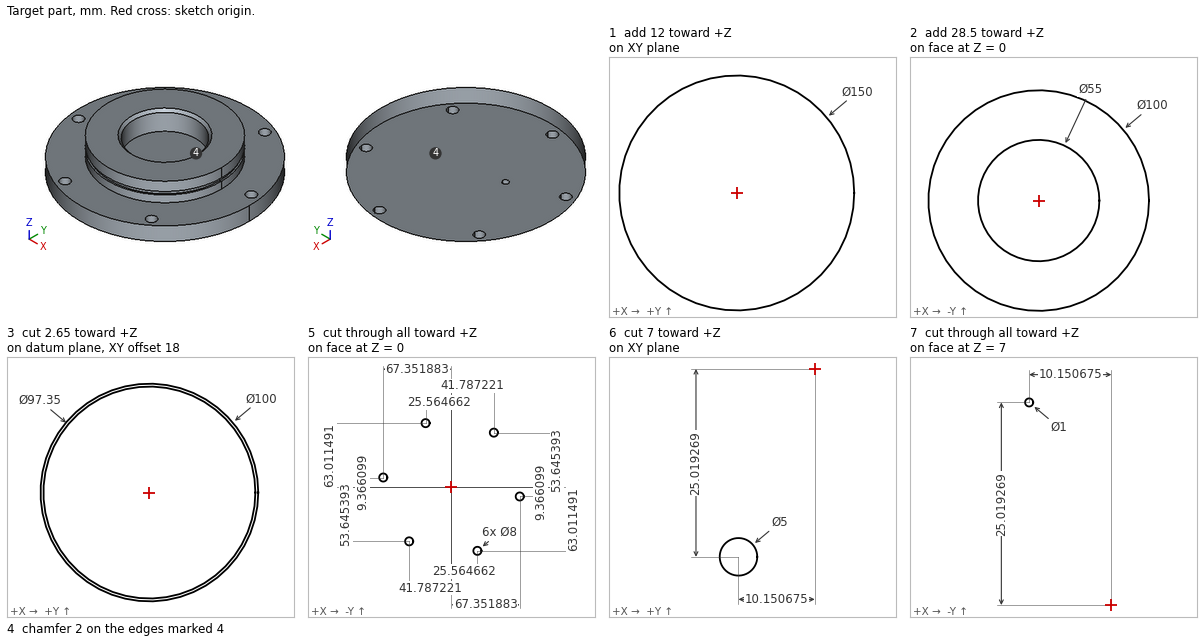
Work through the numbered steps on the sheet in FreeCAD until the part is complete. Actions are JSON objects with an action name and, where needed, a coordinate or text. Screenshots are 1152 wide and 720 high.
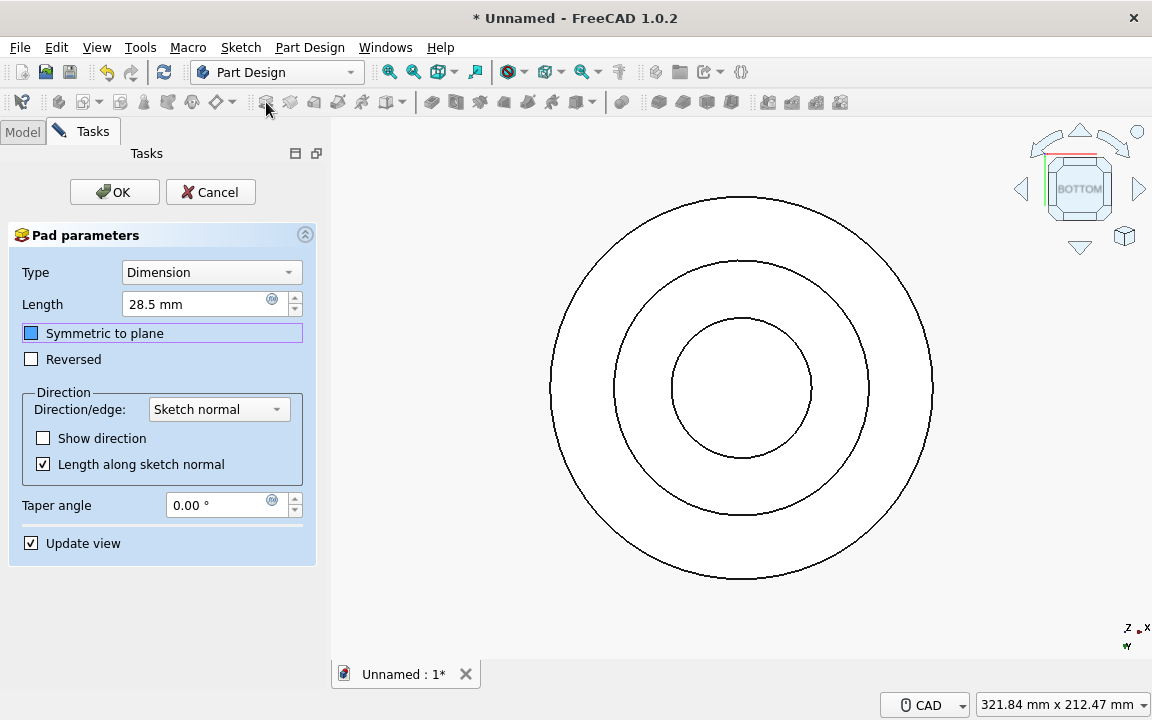
{"action": "left_click", "coordinate": [30, 359]}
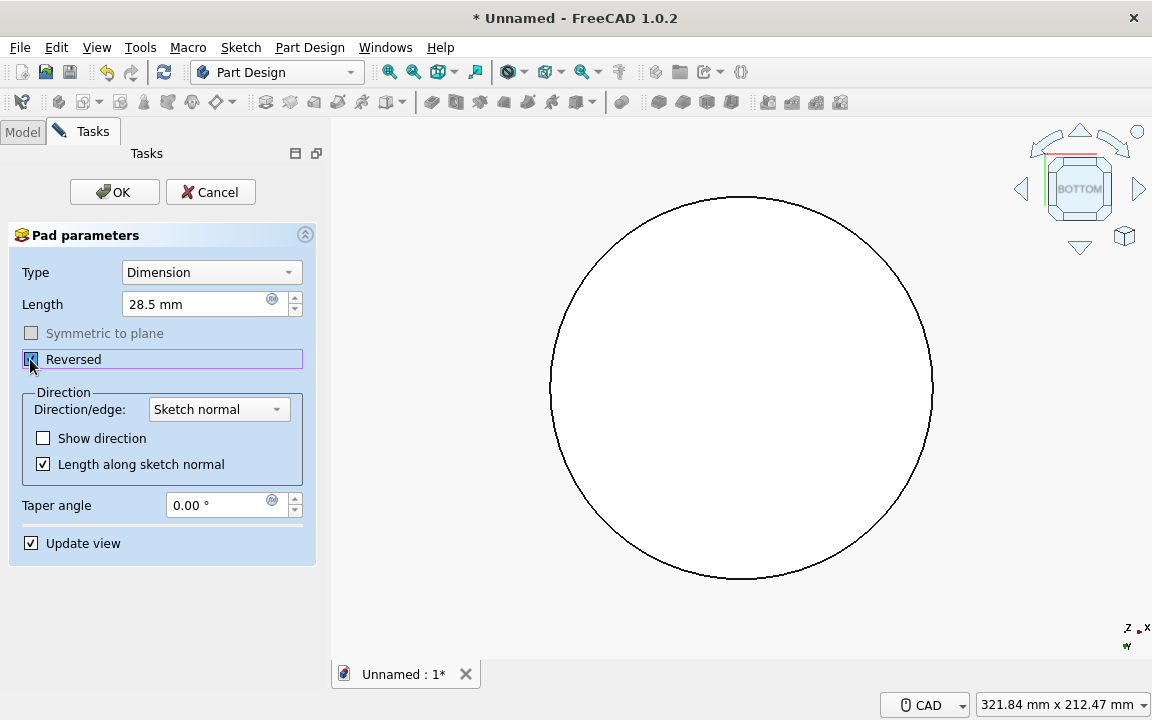
{"action": "left_click", "coordinate": [115, 192]}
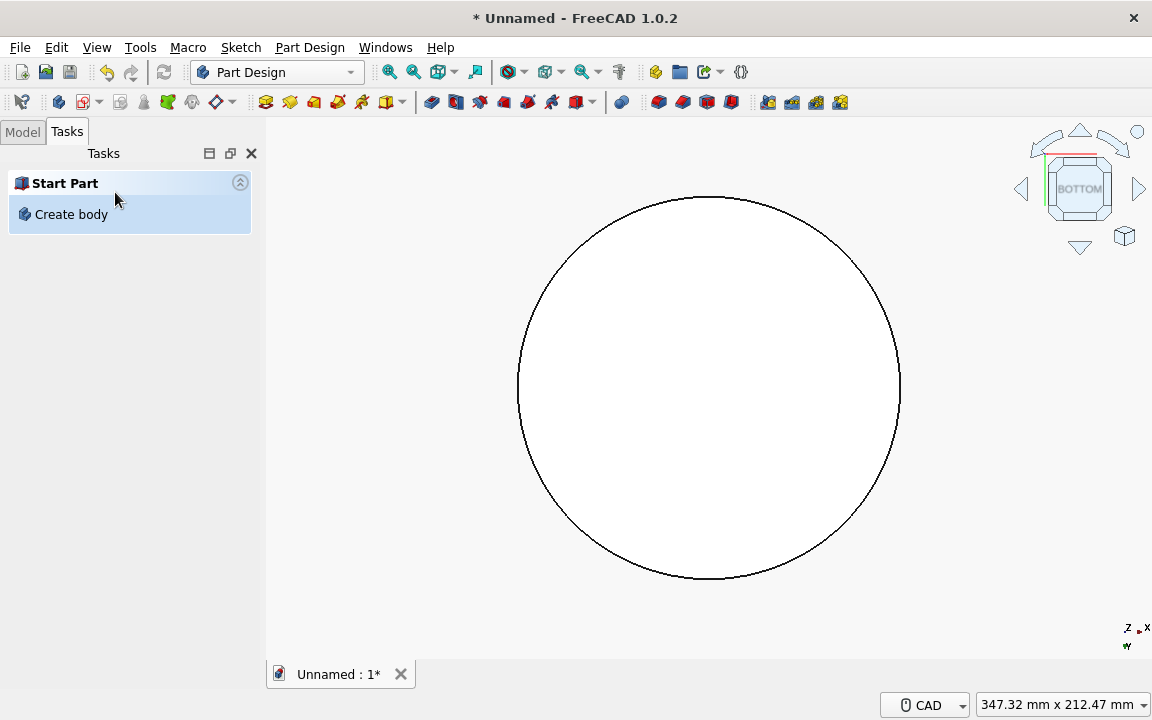
{"action": "left_click", "coordinate": [23, 131]}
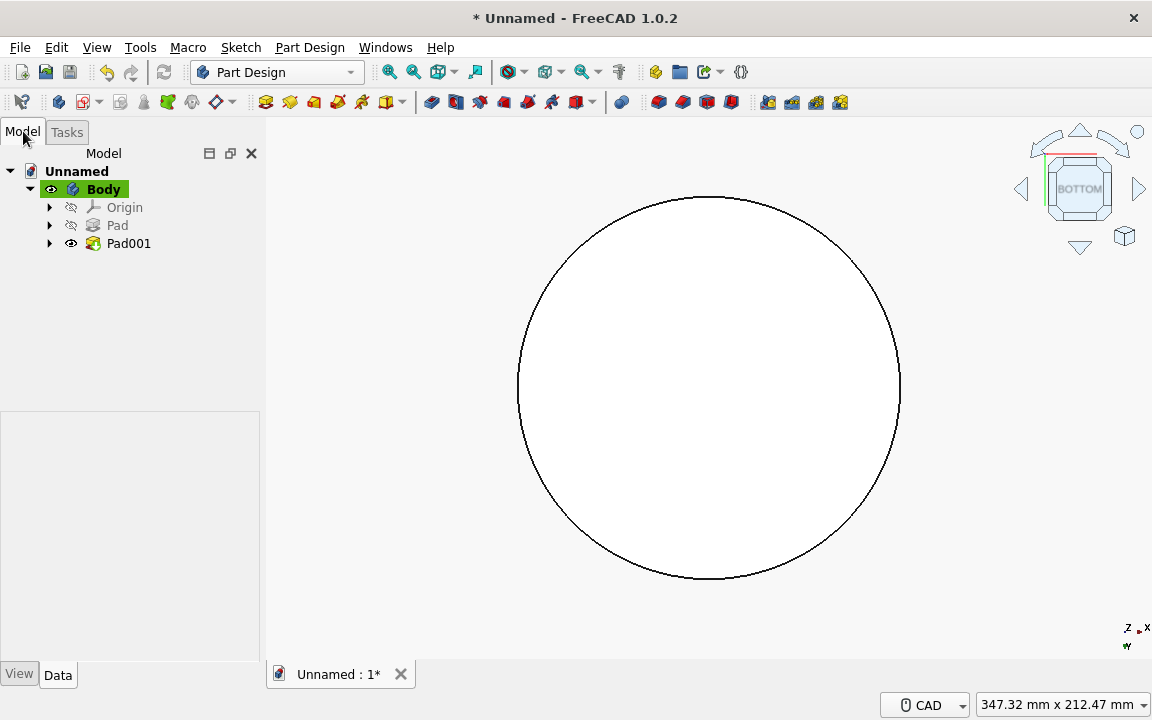
{"action": "left_click", "coordinate": [50, 207]}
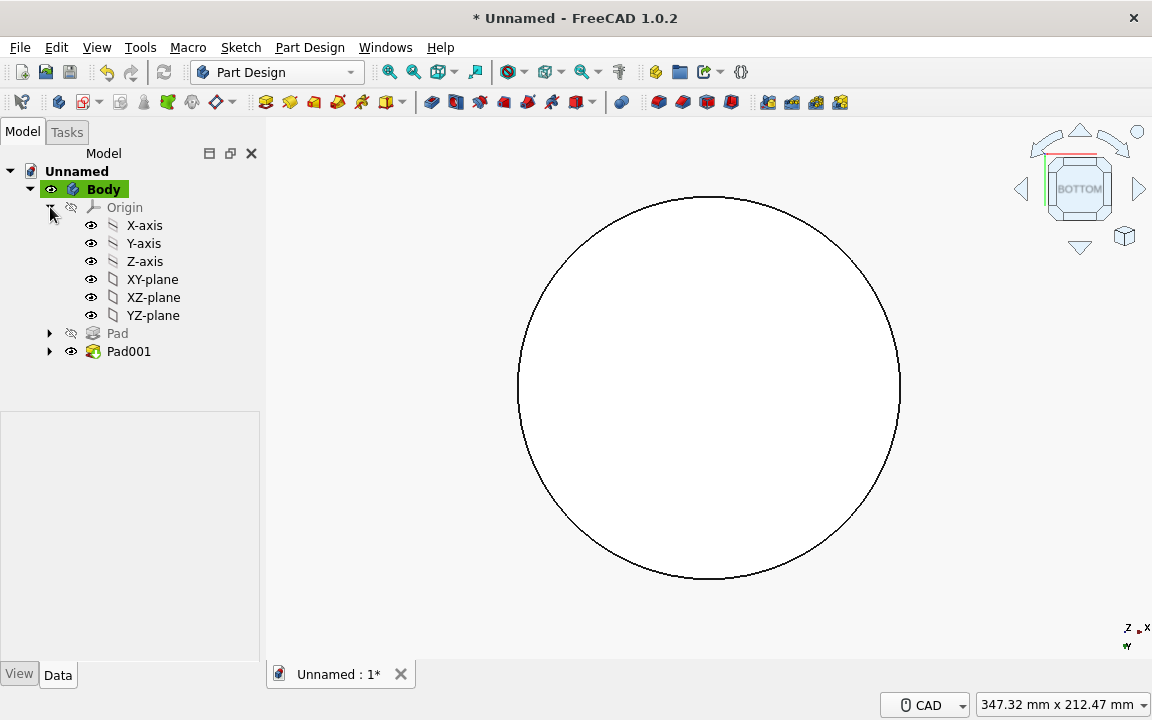
{"action": "left_click", "coordinate": [136, 279]}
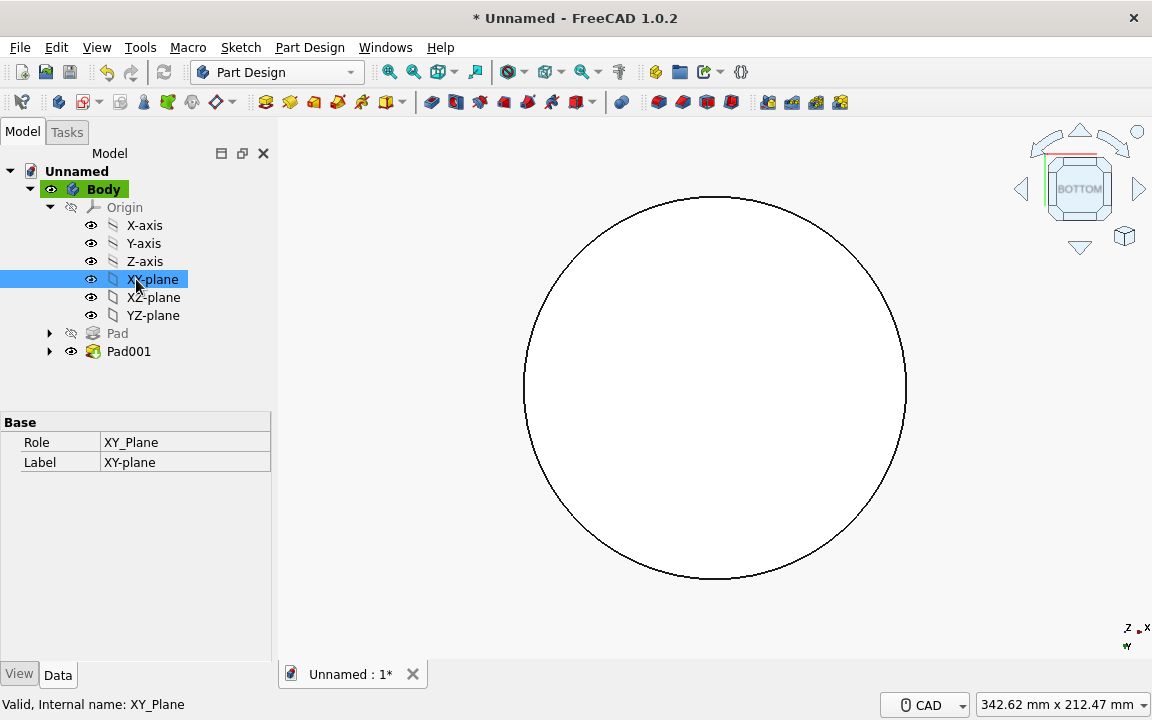
{"action": "left_click", "coordinate": [216, 102]}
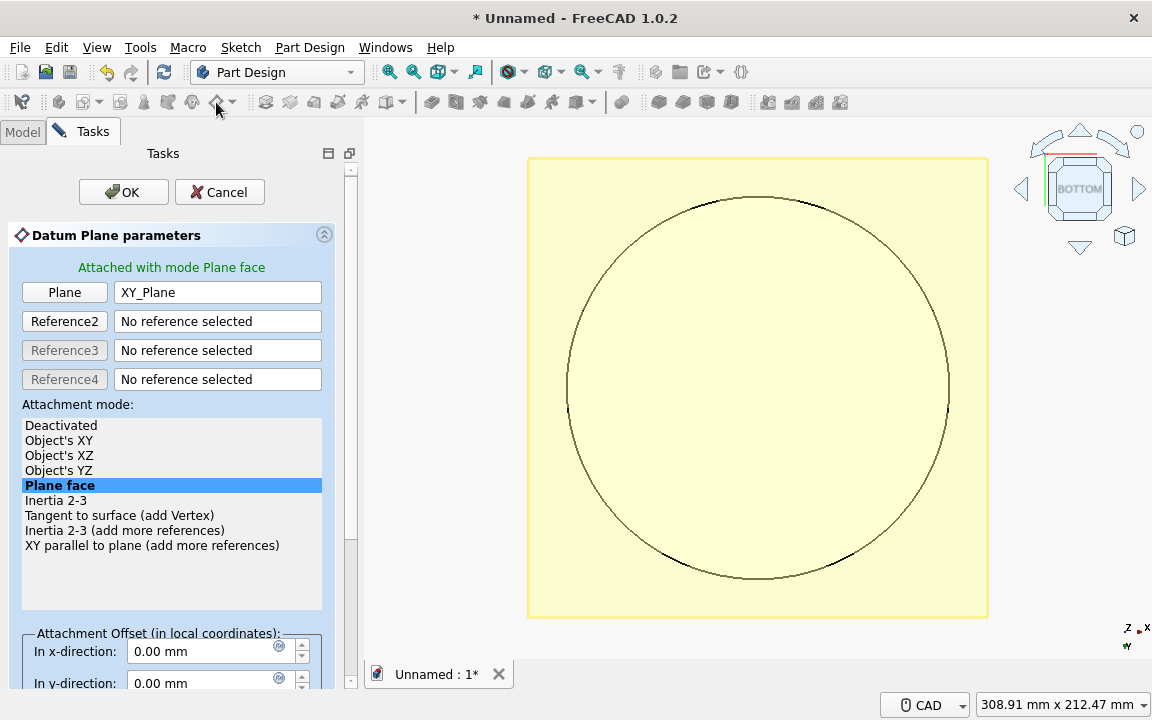
{"action": "scroll", "coordinate": [351, 426], "scroll_direction": "down", "scroll_amount": 2}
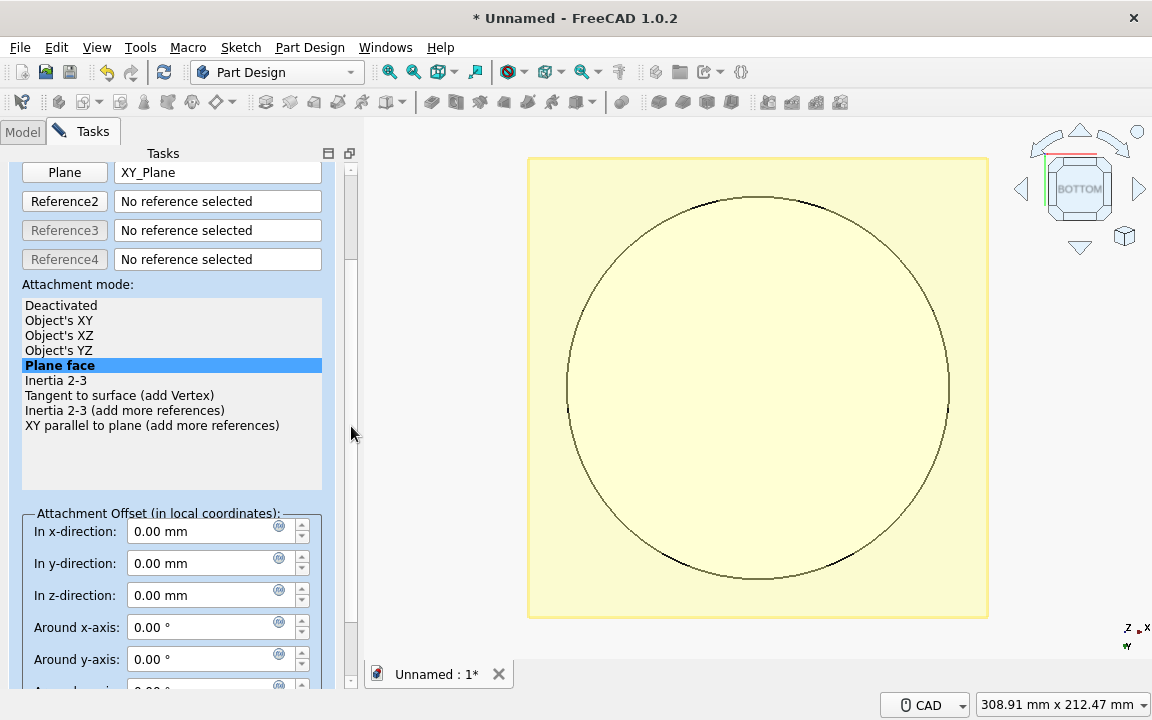
{"action": "triple_click", "coordinate": [210, 595]}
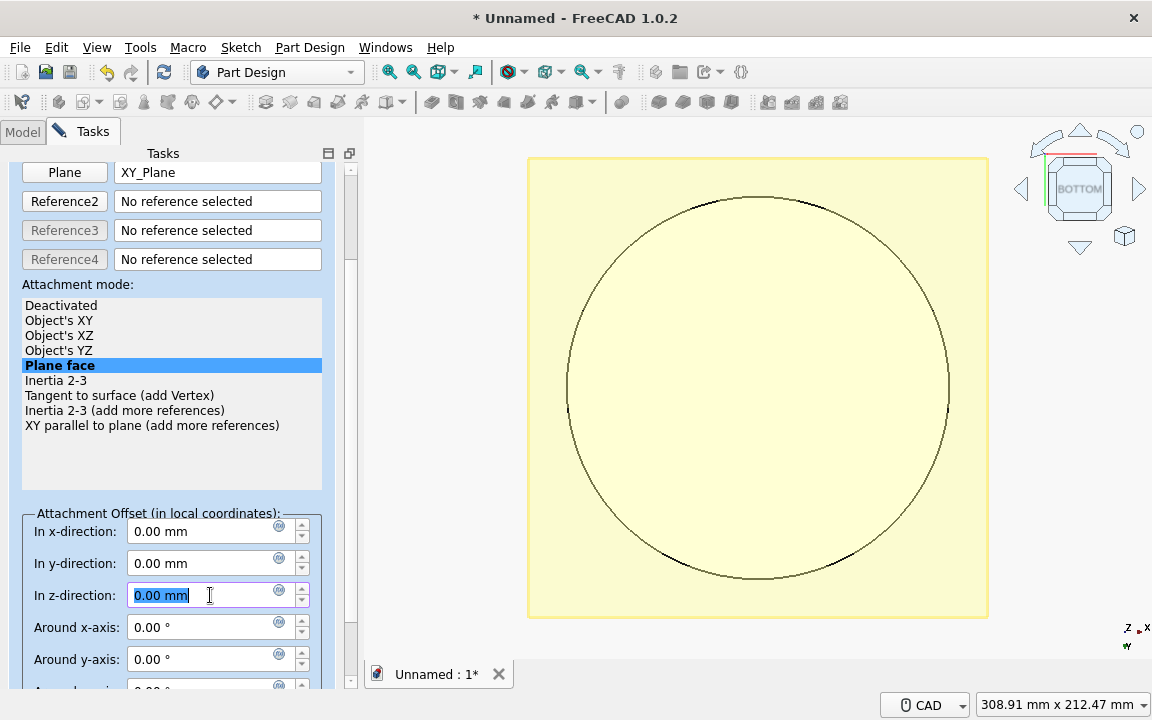
{"action": "type", "text": "18"}
{"action": "key", "text": "Tab"}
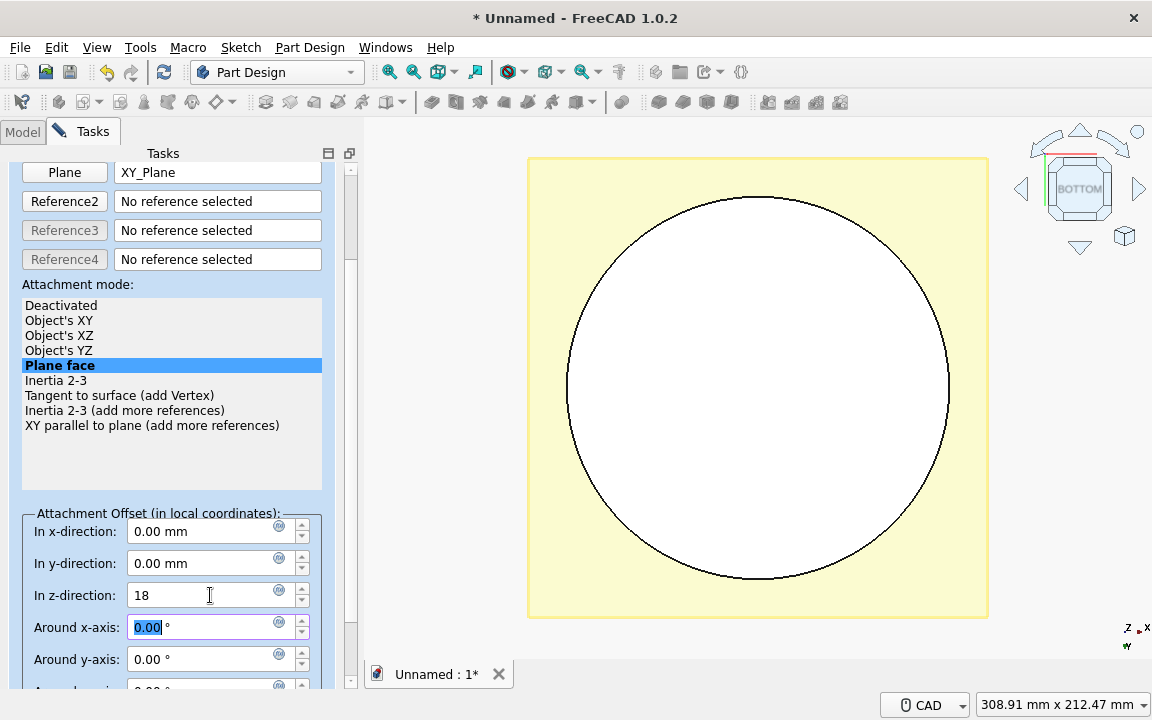
{"action": "scroll", "coordinate": [351, 426], "scroll_direction": "up", "scroll_amount": 3}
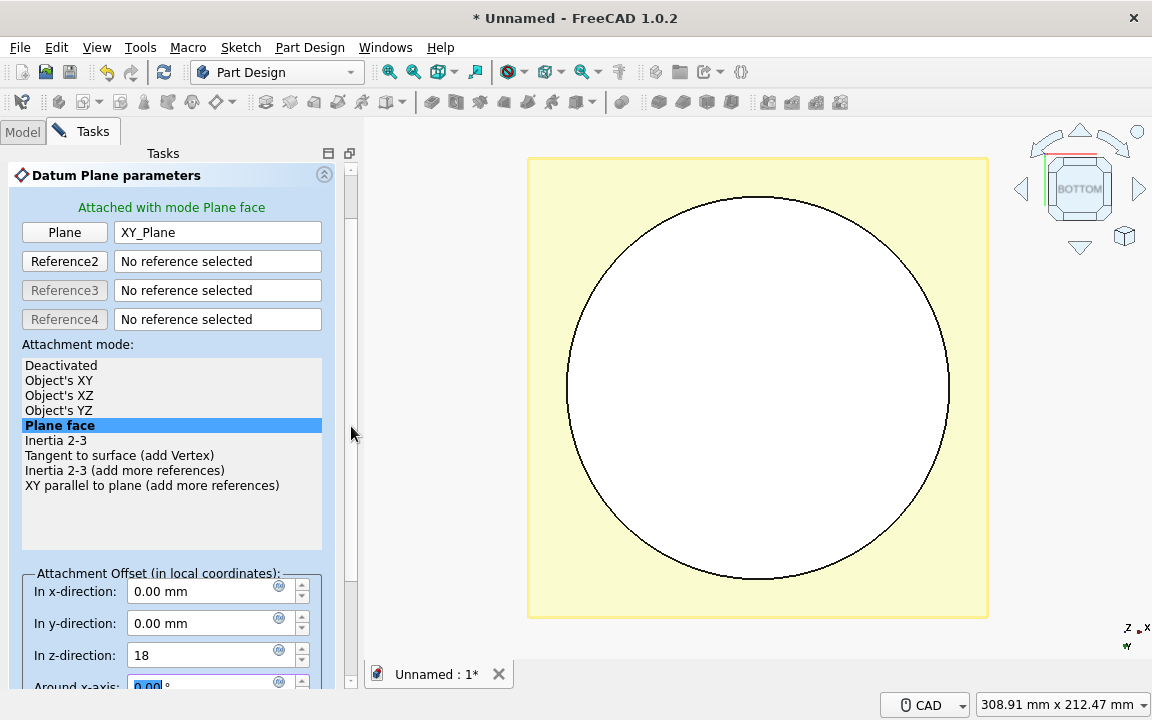
{"action": "left_click", "coordinate": [124, 192]}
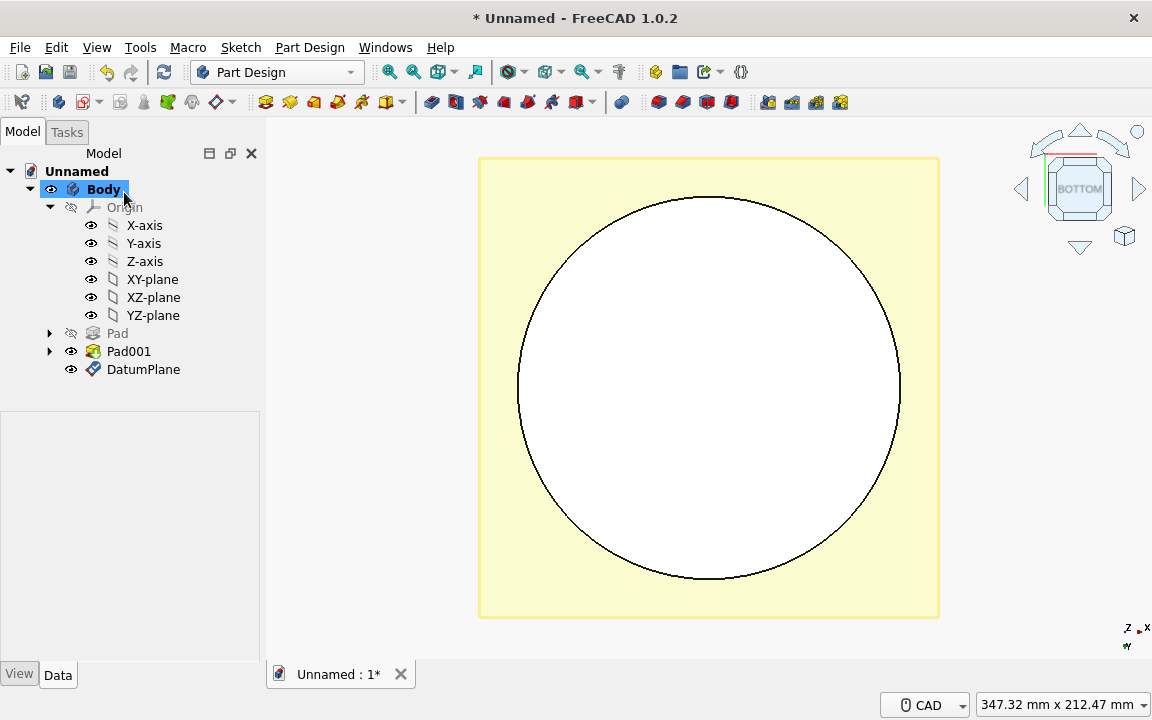
{"action": "left_click", "coordinate": [116, 369]}